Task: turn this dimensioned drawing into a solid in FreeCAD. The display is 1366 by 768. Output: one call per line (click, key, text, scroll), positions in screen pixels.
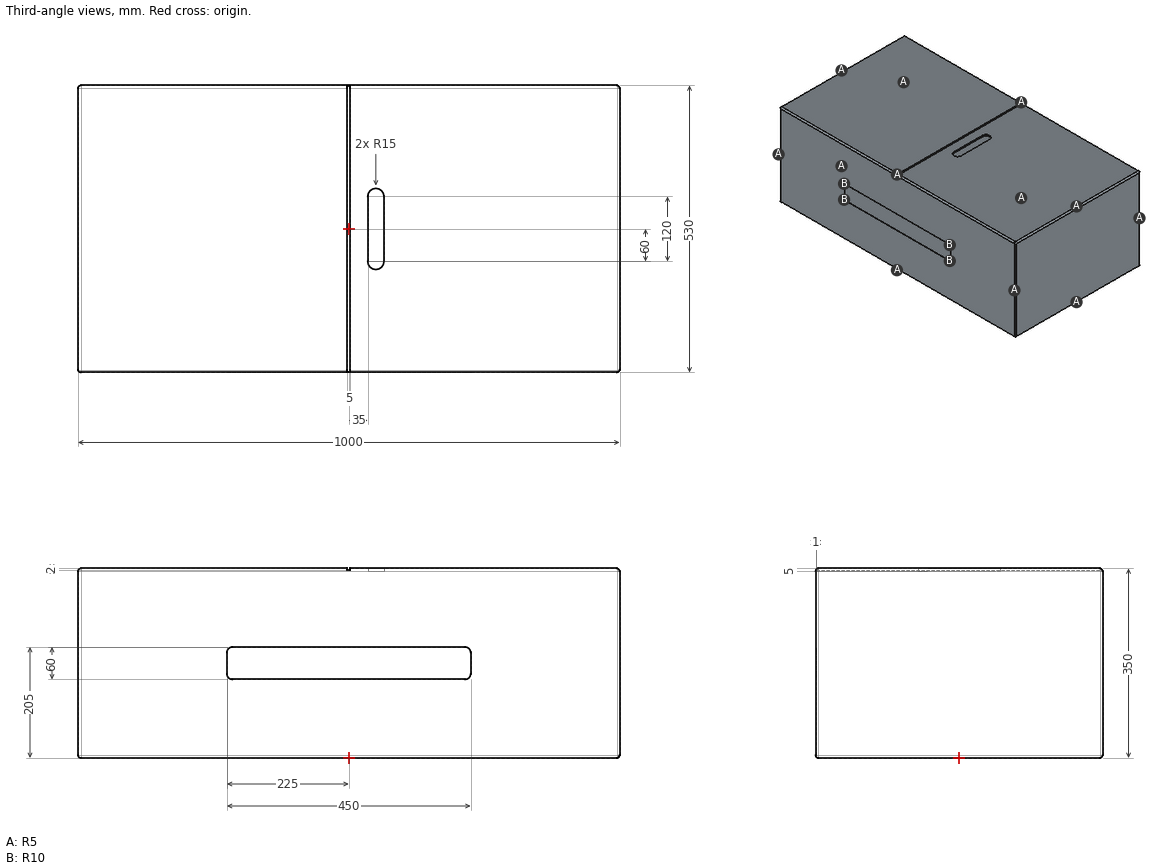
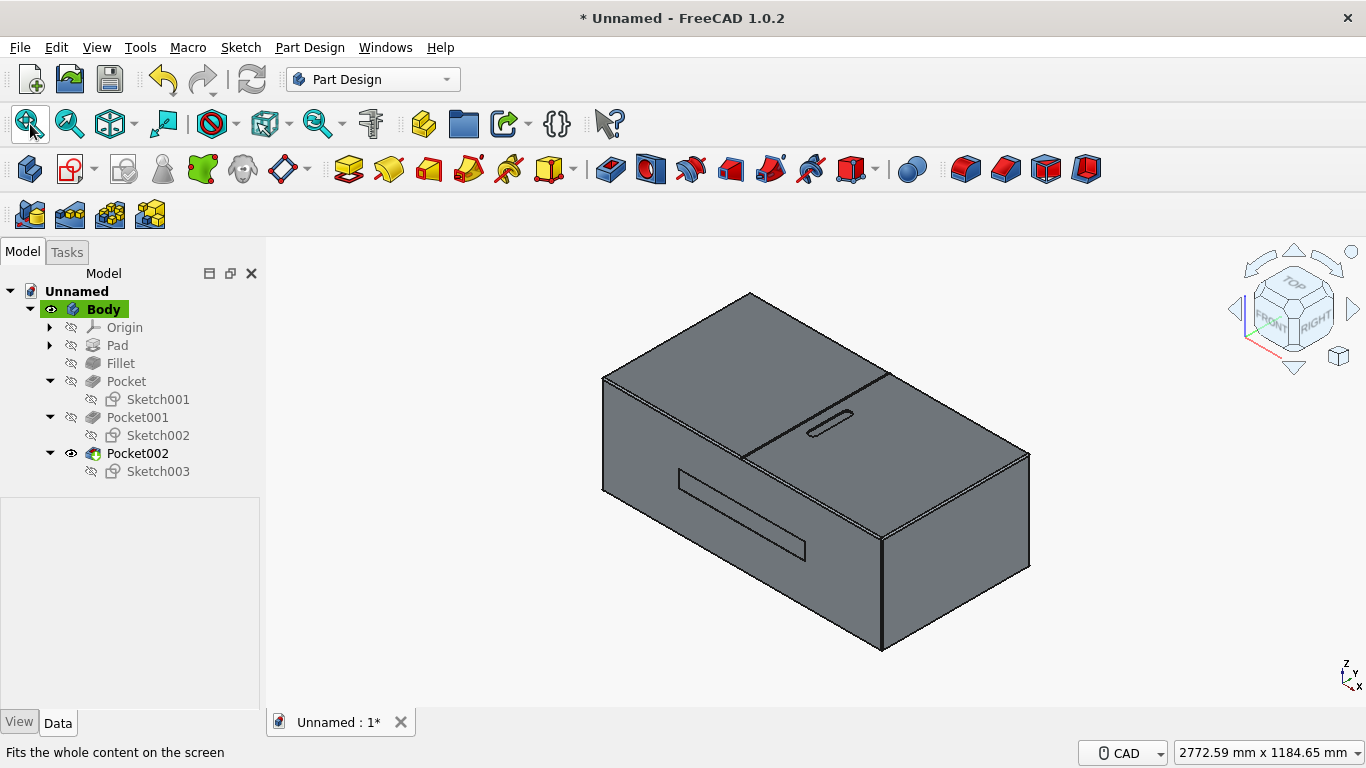
key(2)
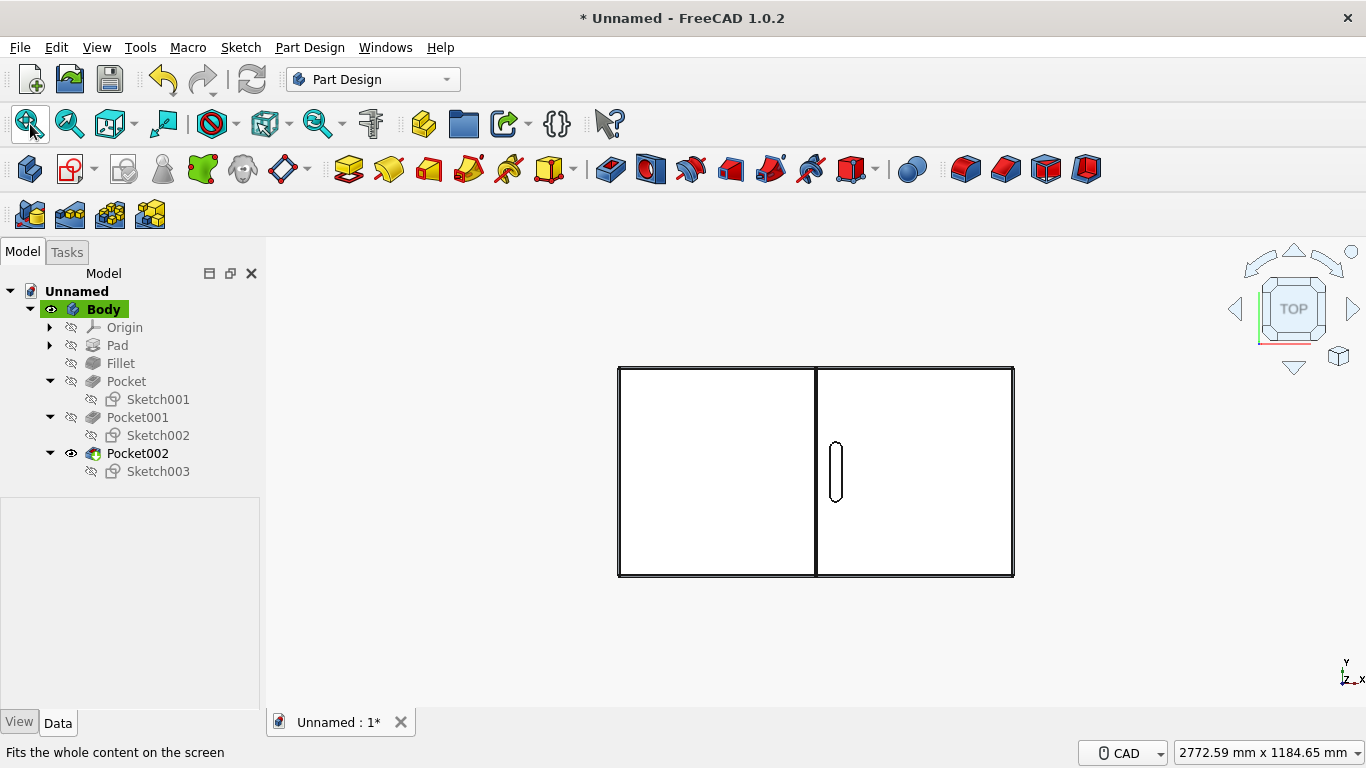
click(30, 124)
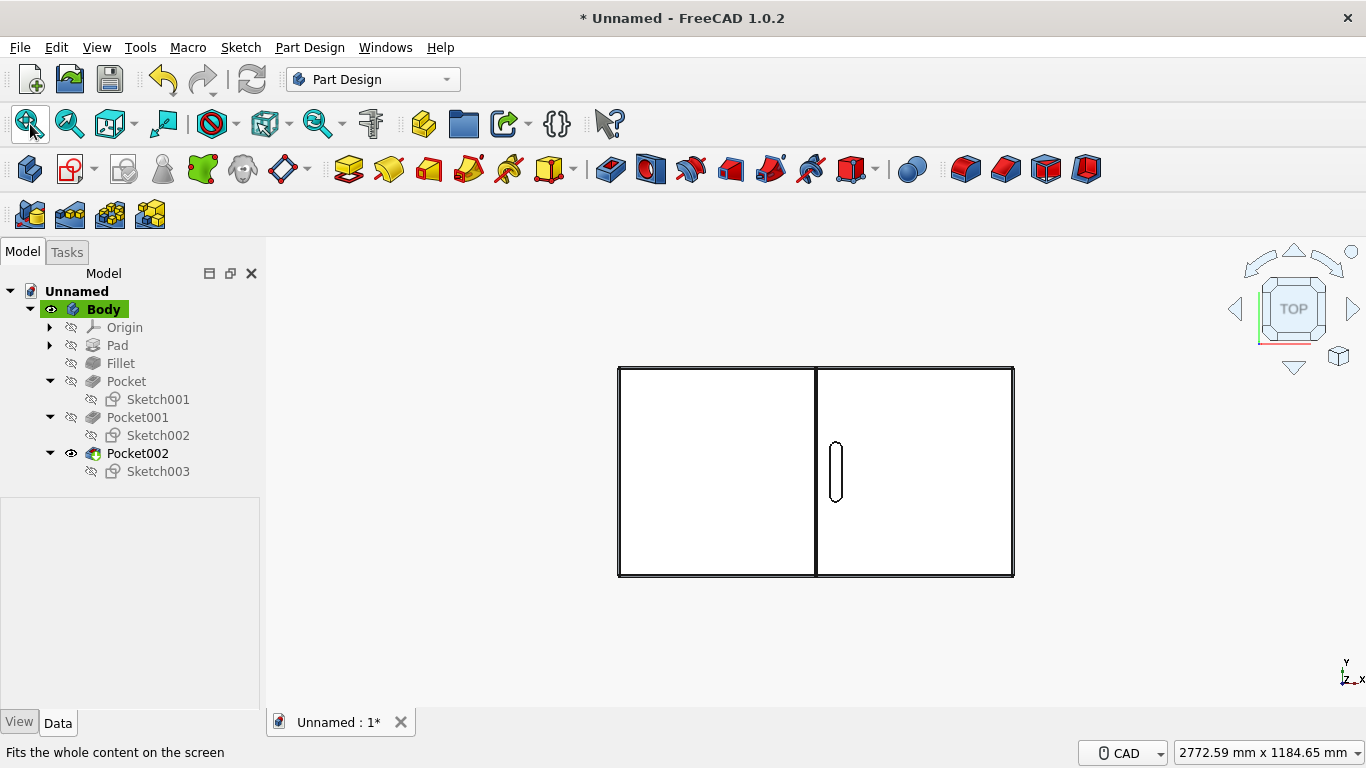
scroll(905, 576, up, 15)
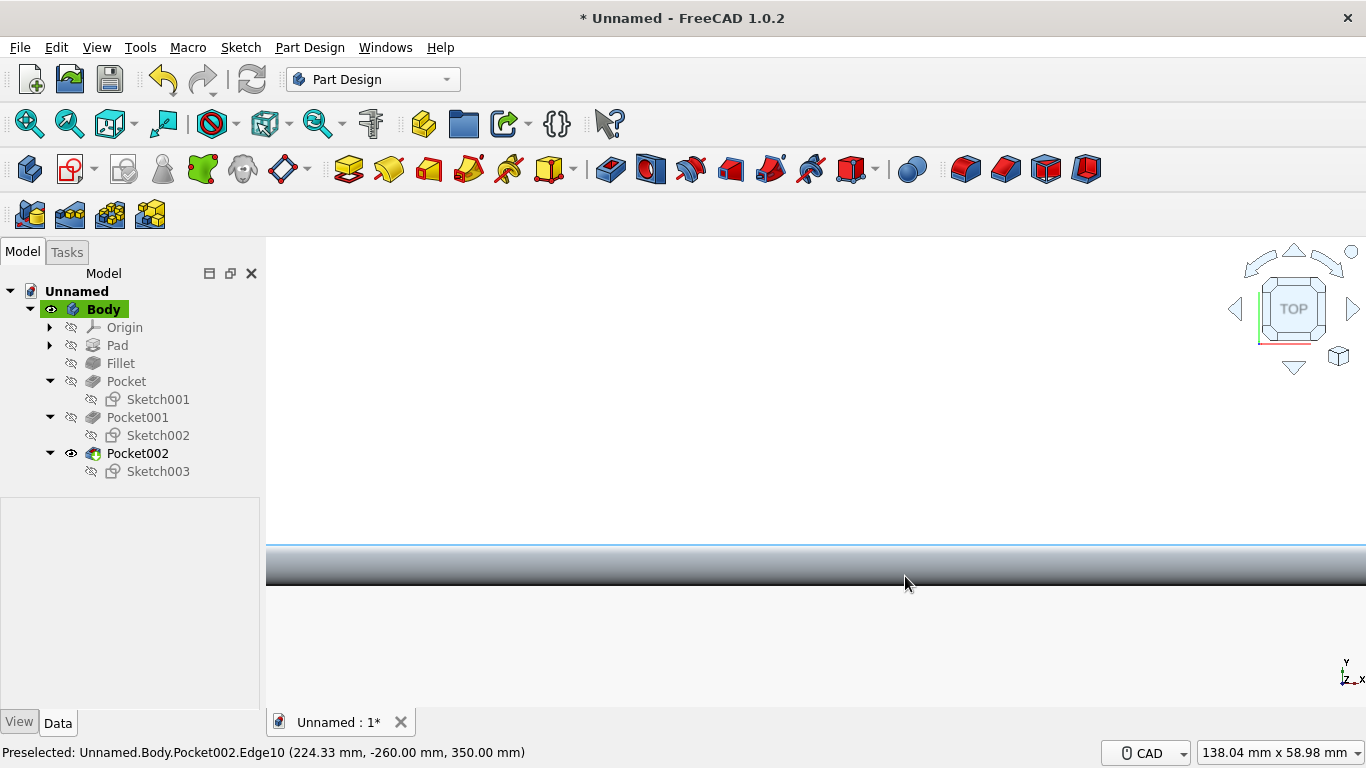
scroll(899, 580, up, 9)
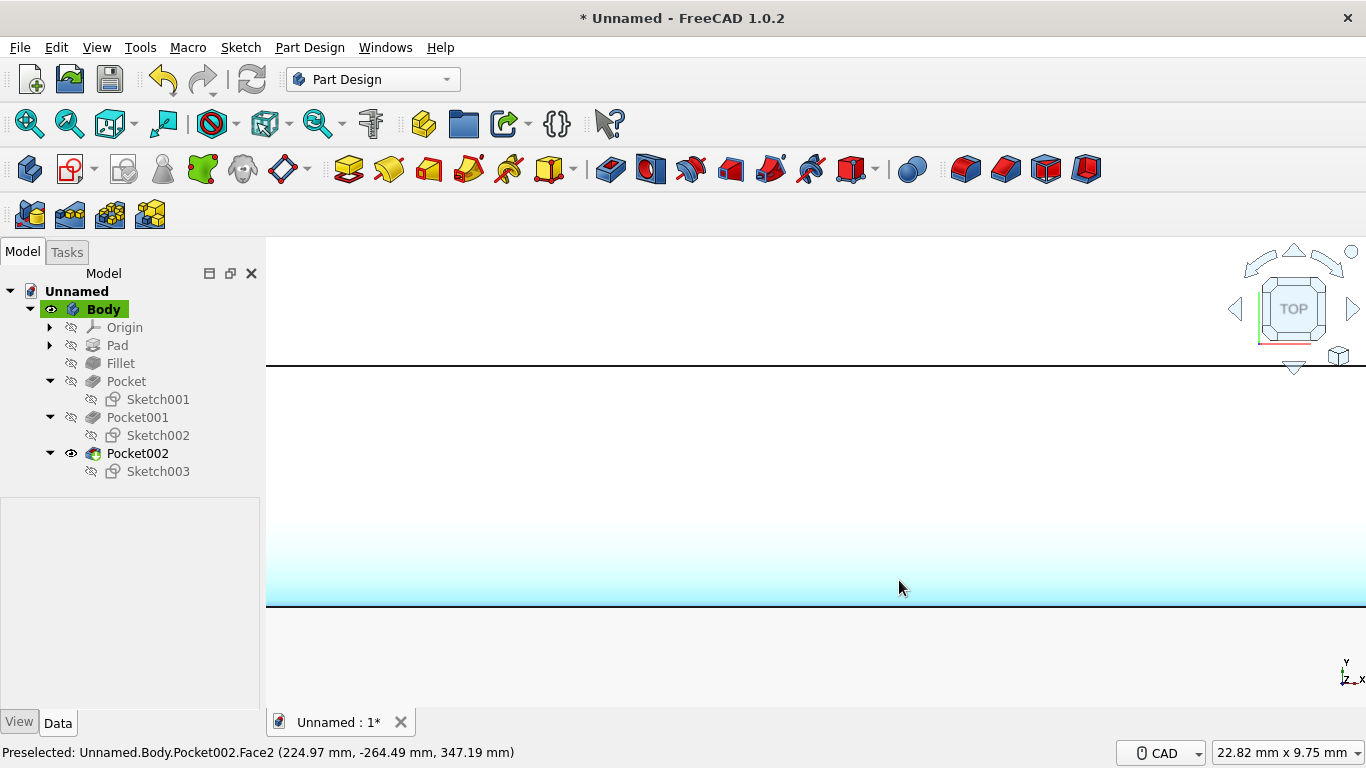
click(30, 124)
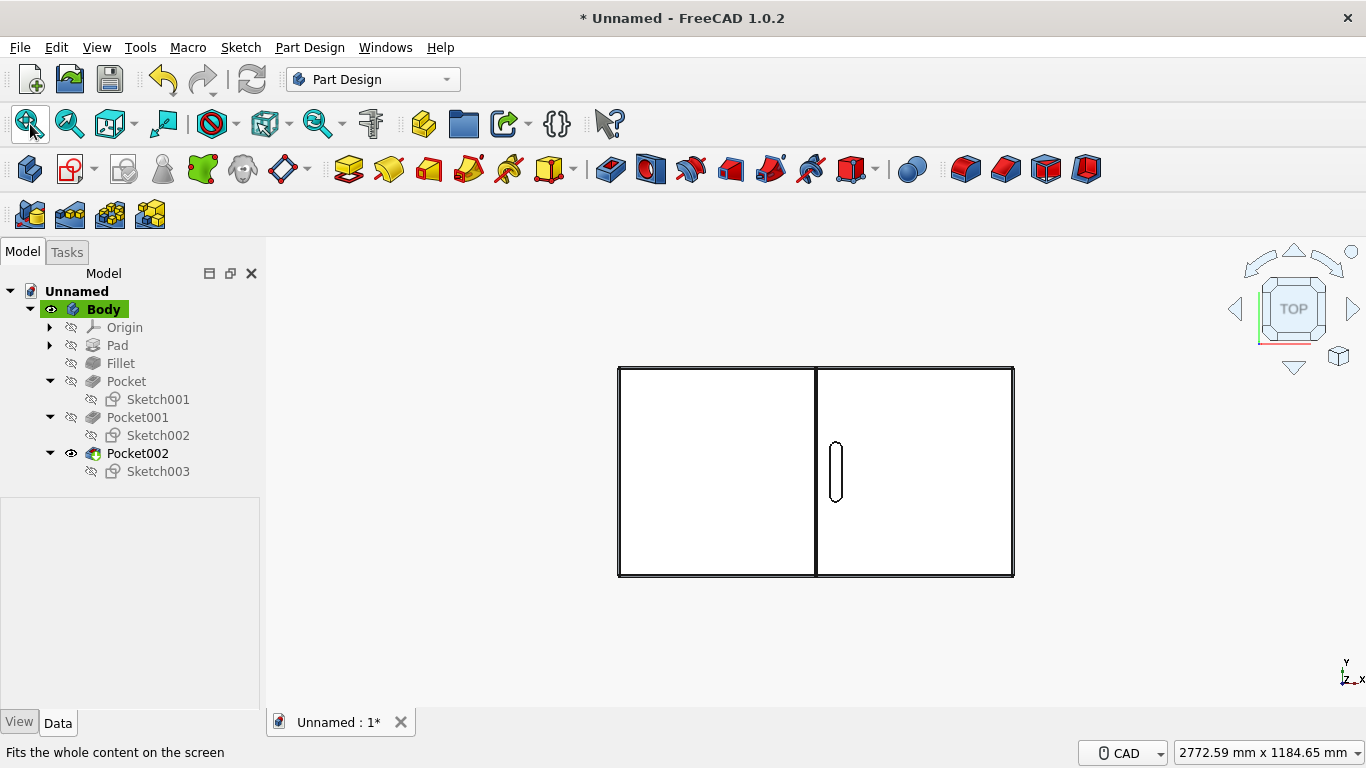
key(0)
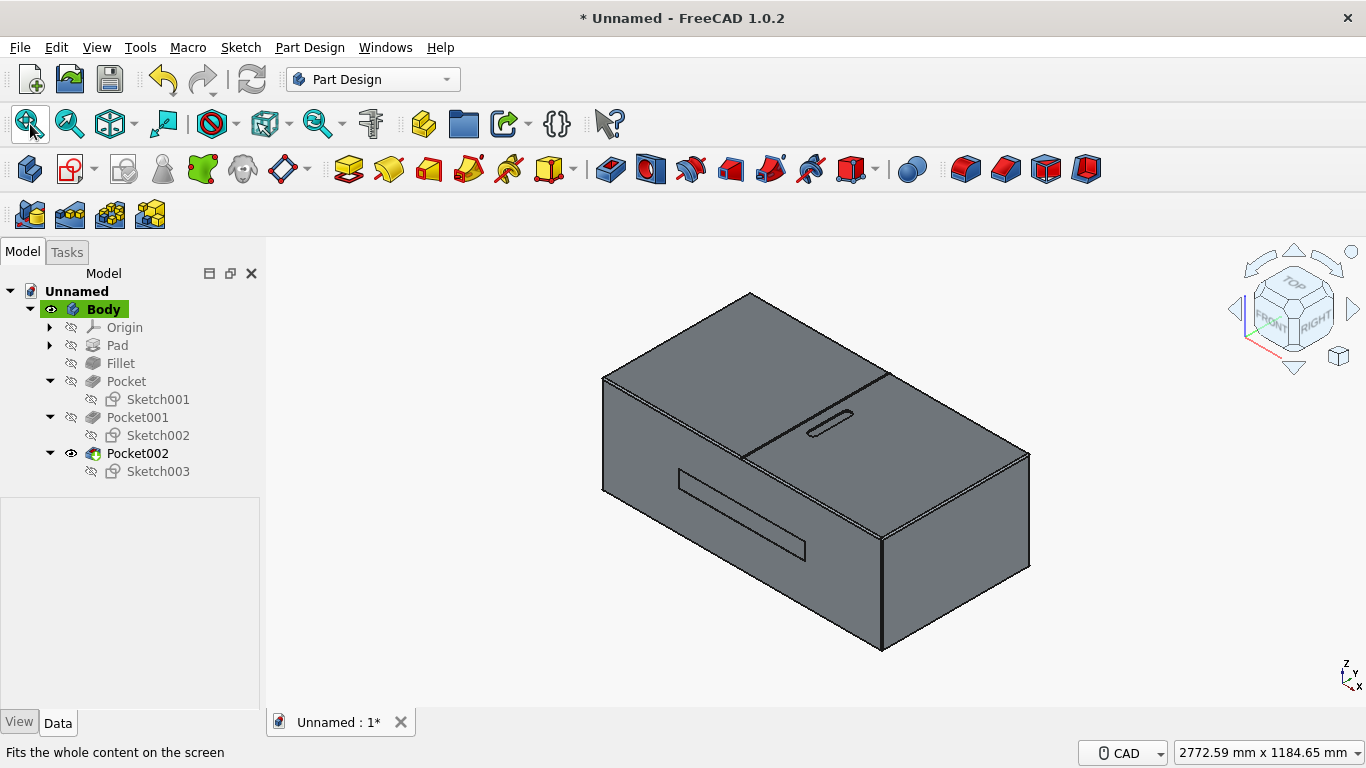
scroll(805, 541, up, 15)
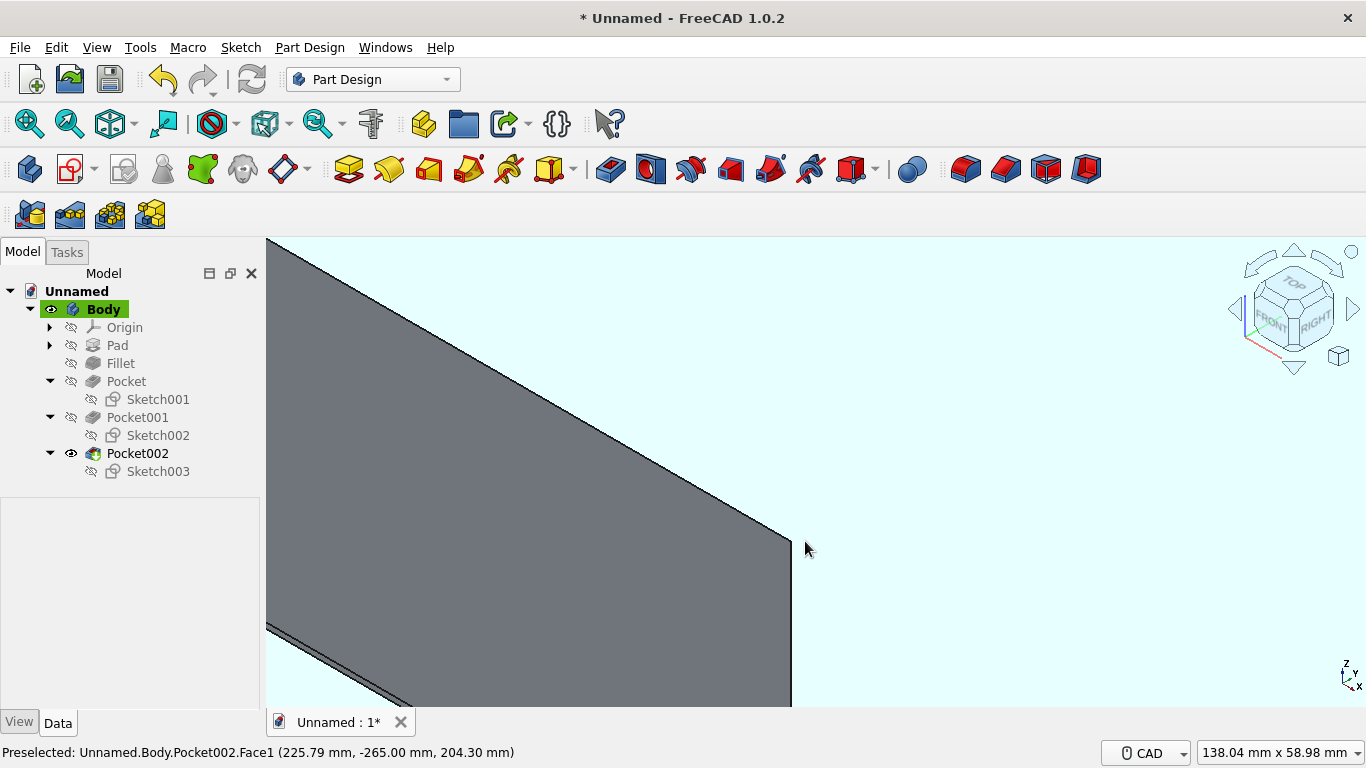
scroll(794, 539, up, 9)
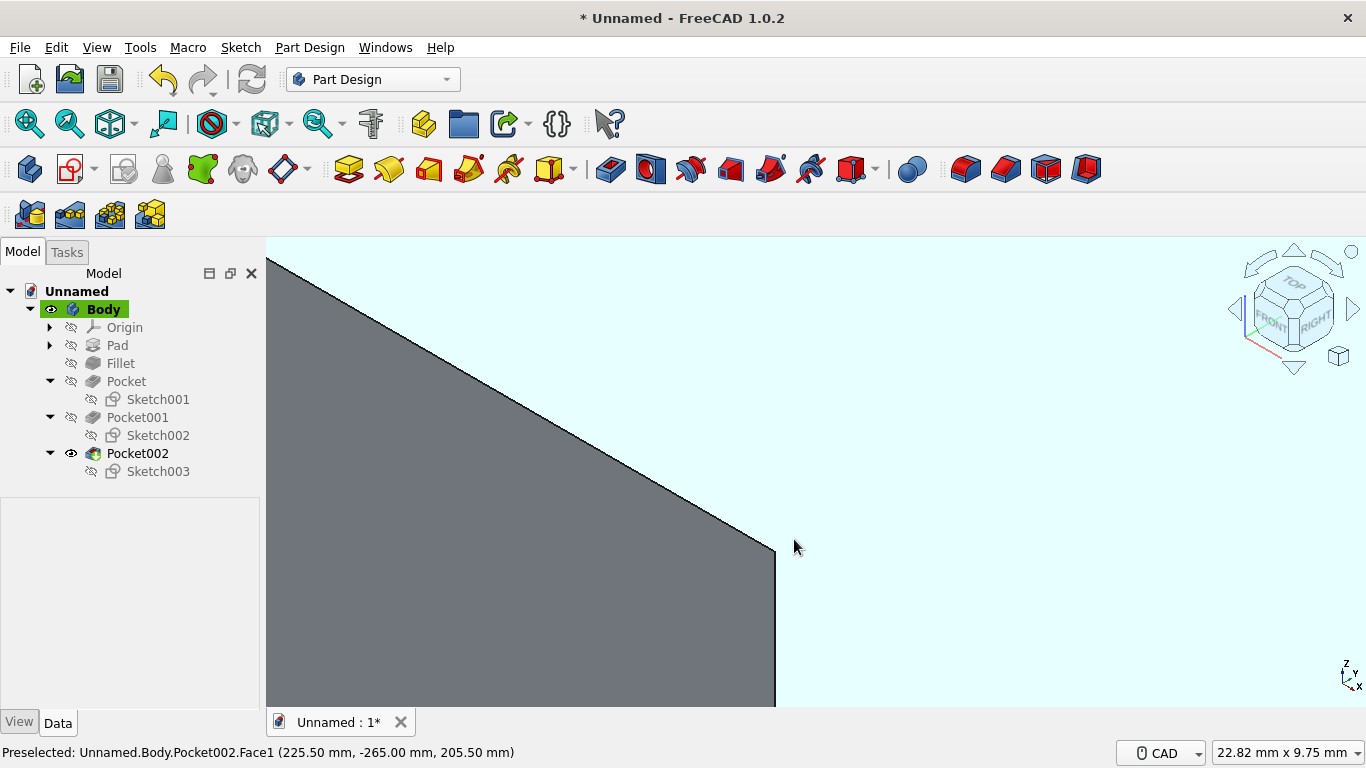
click(30, 124)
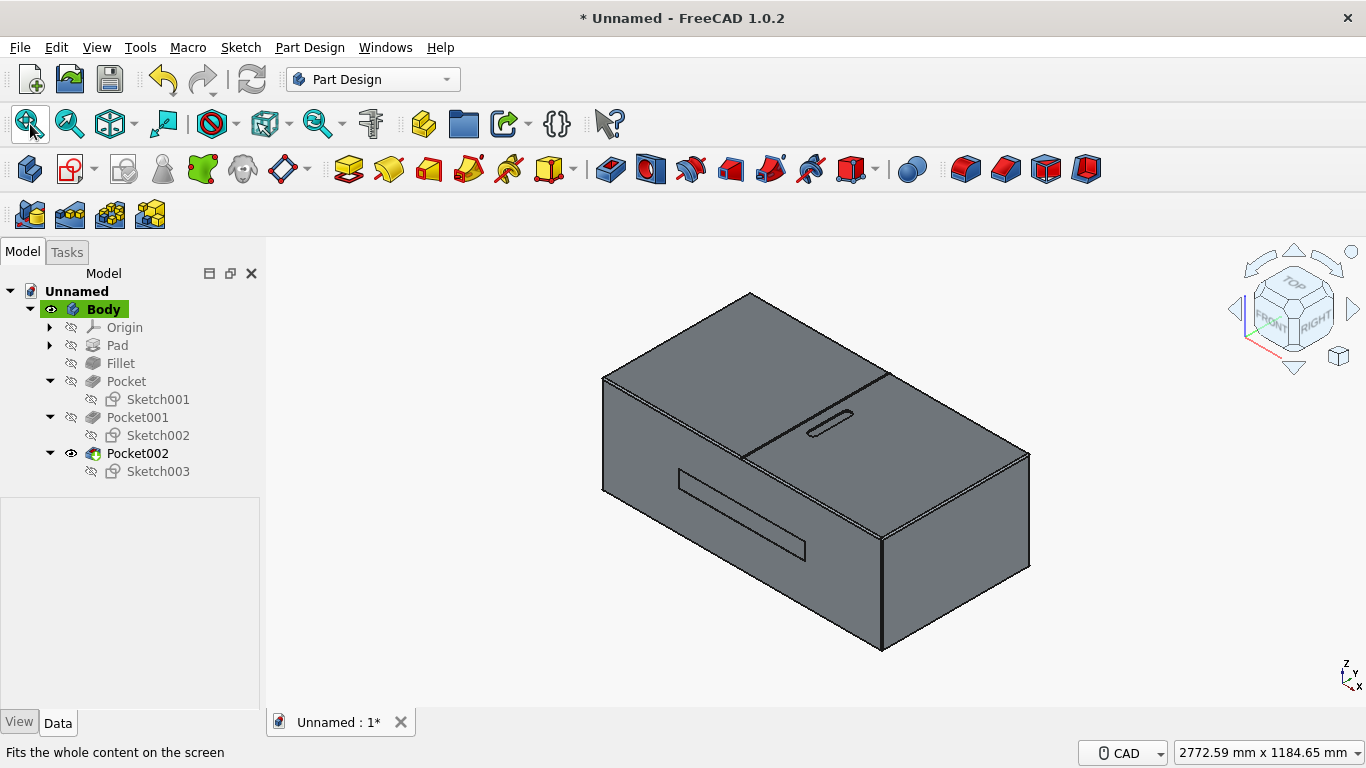
key(1)